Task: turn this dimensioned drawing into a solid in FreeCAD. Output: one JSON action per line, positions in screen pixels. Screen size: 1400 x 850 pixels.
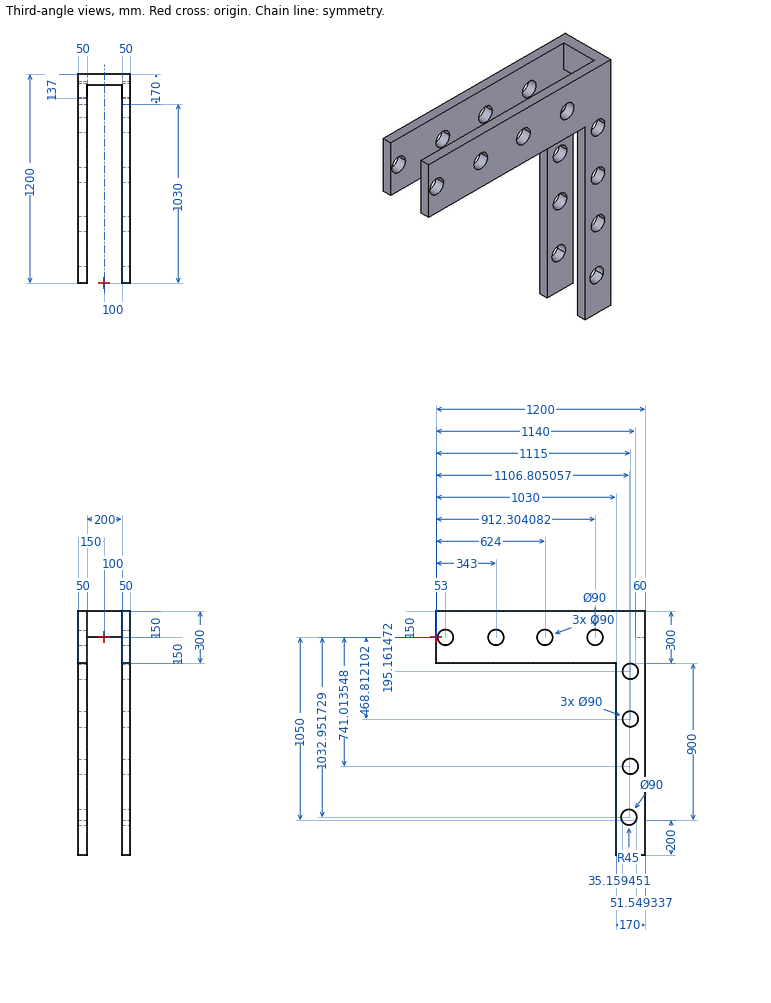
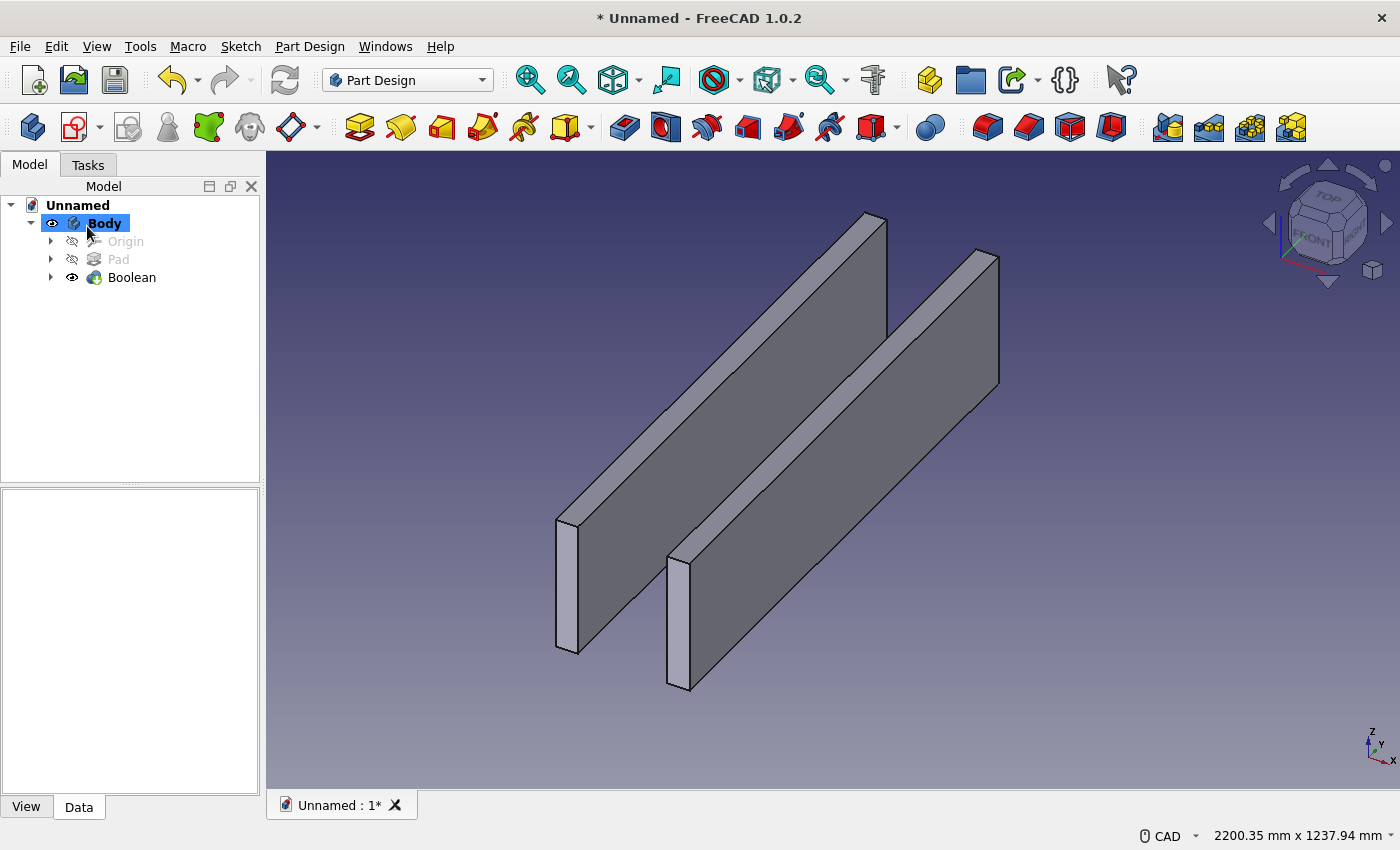
{"action": "left_click", "coordinate": [51, 241]}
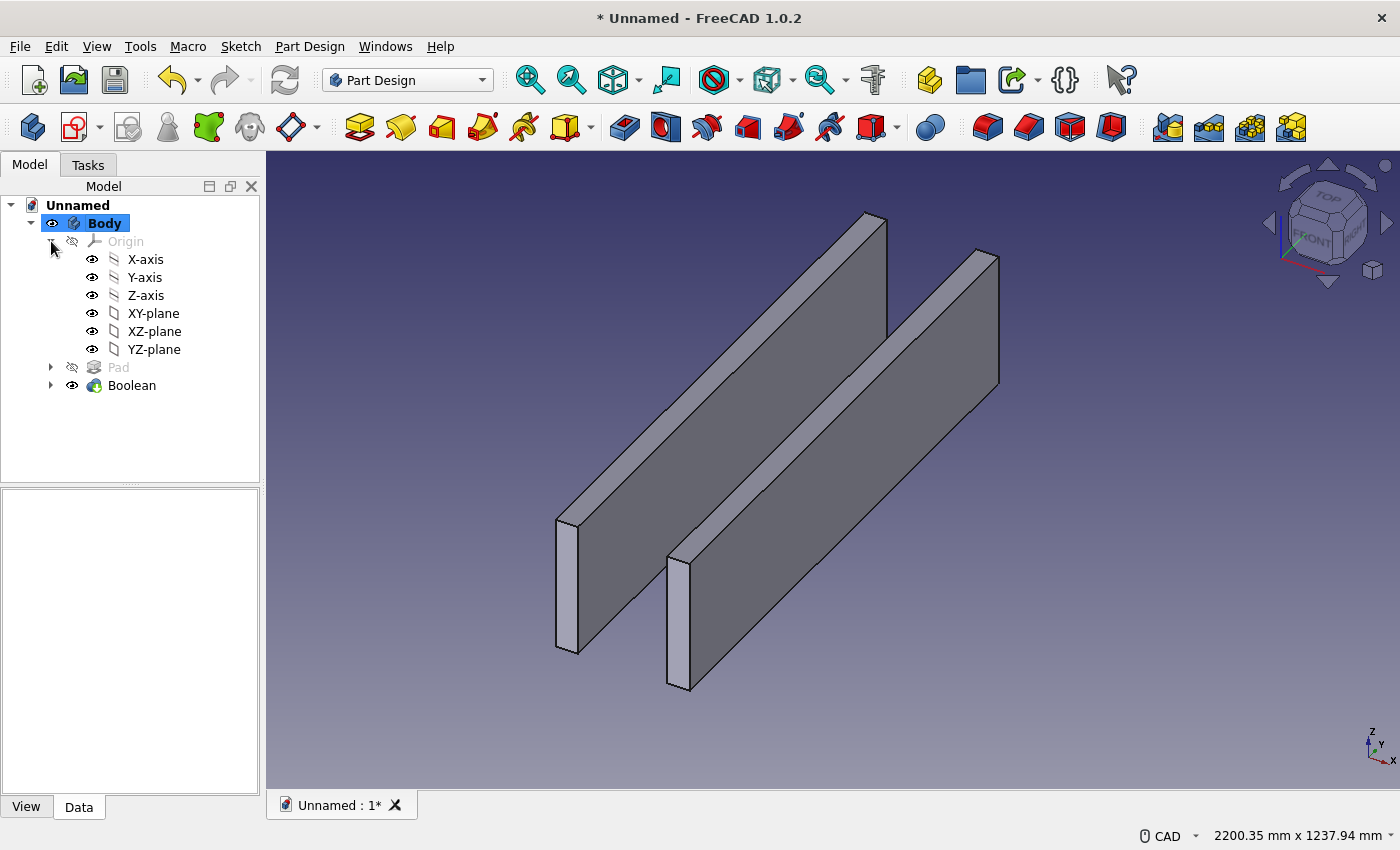
{"action": "left_click", "coordinate": [137, 349]}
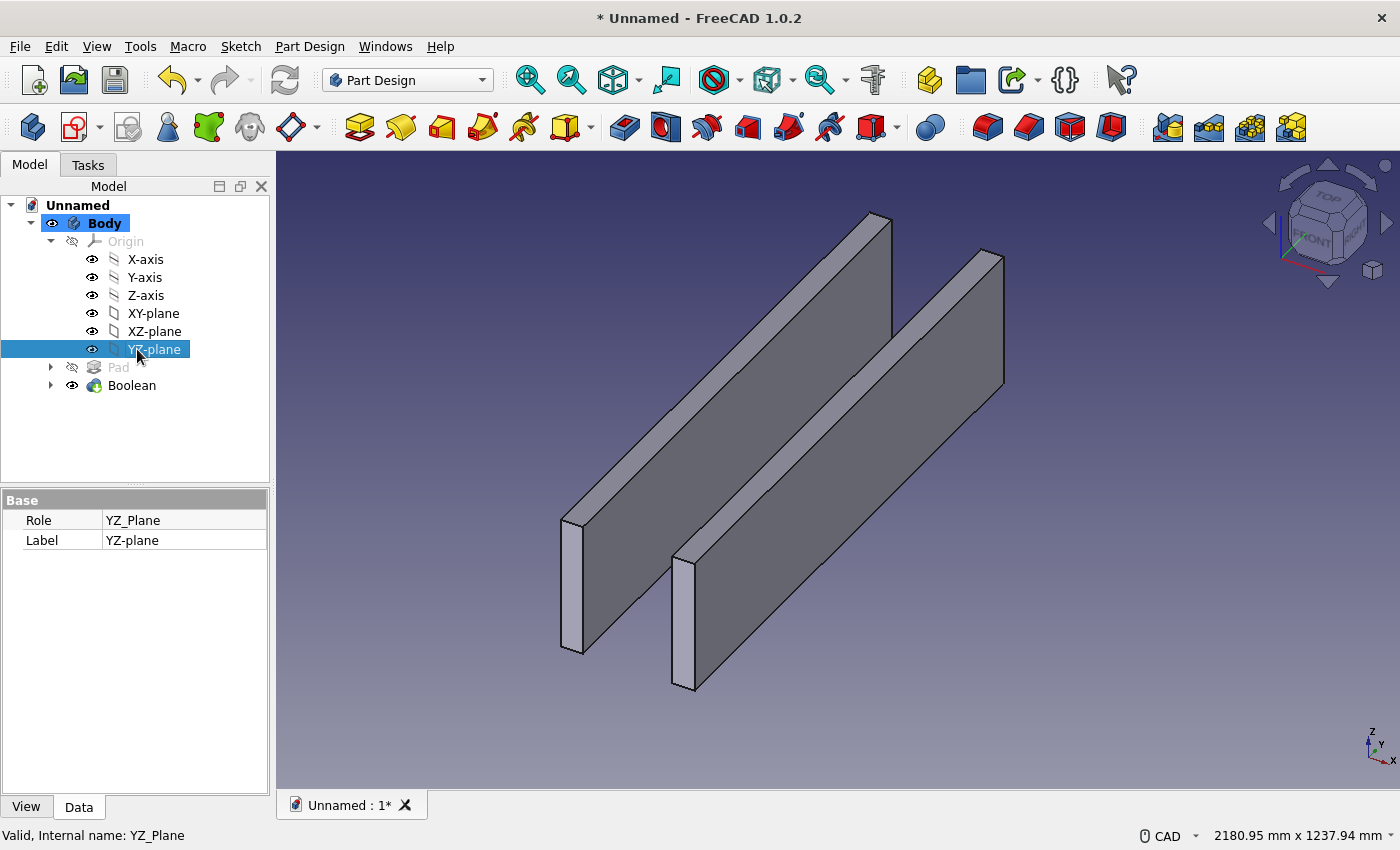
{"action": "left_click", "coordinate": [290, 128]}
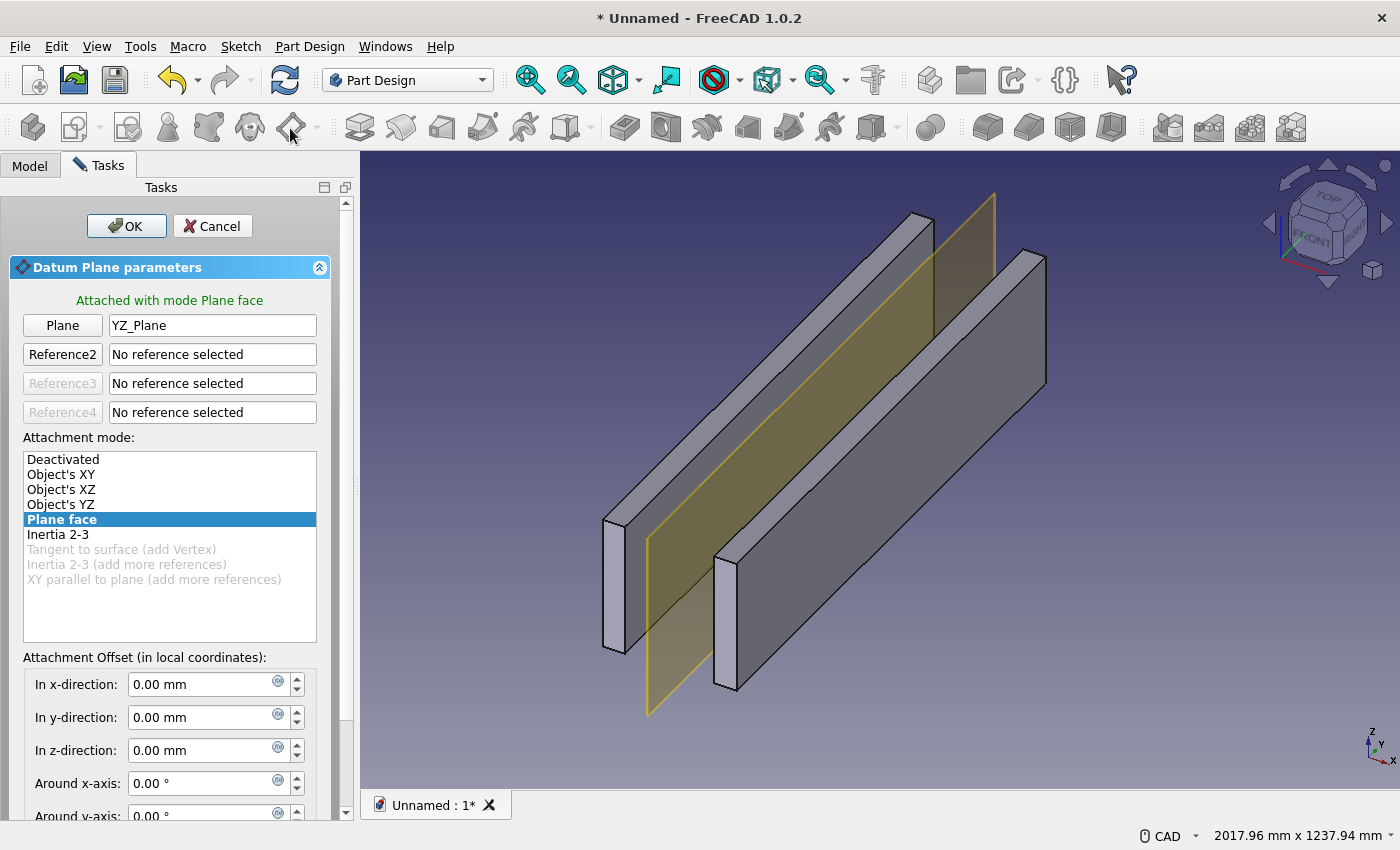
{"action": "triple_click", "coordinate": [210, 750]}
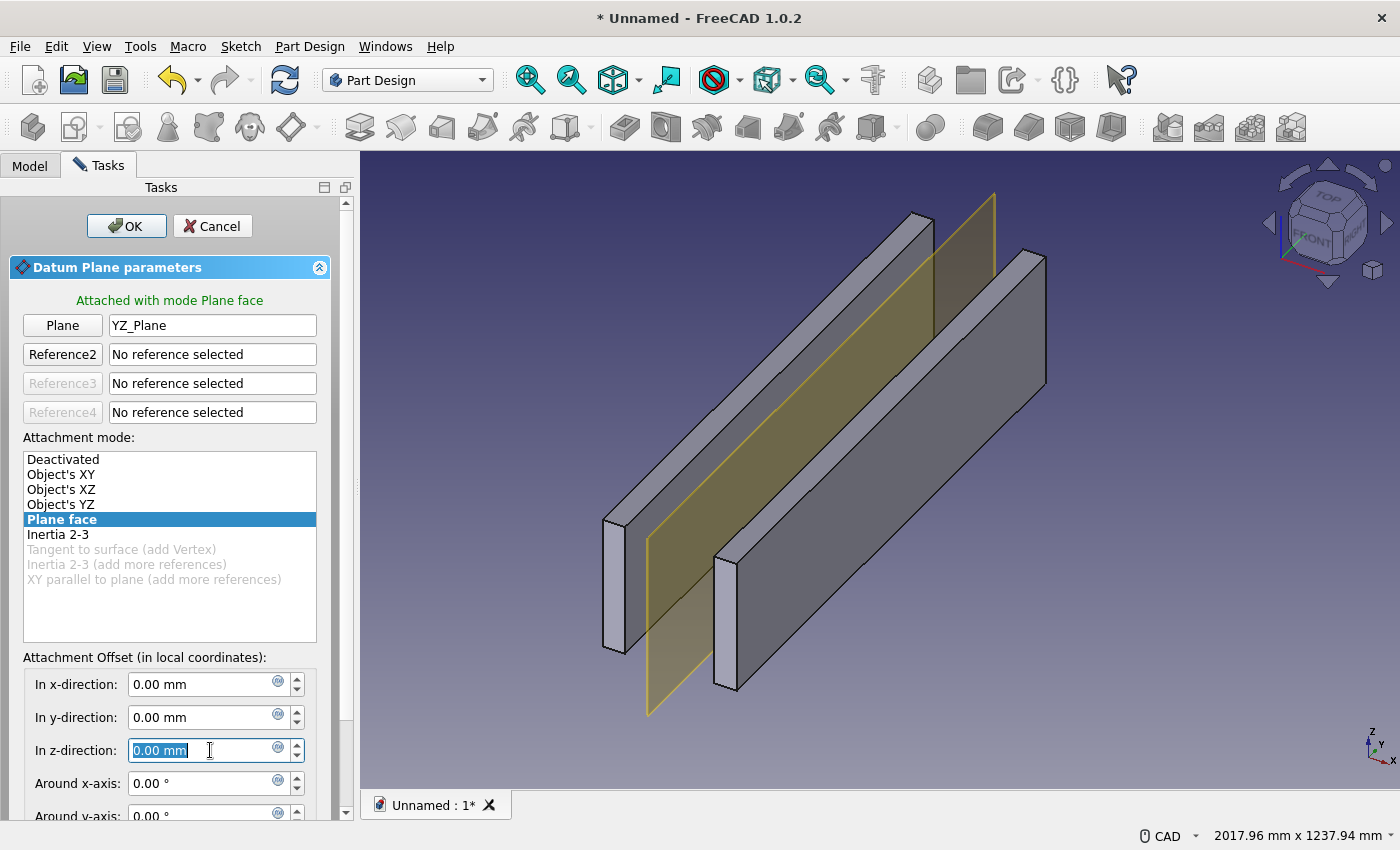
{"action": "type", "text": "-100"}
{"action": "key", "text": "Tab"}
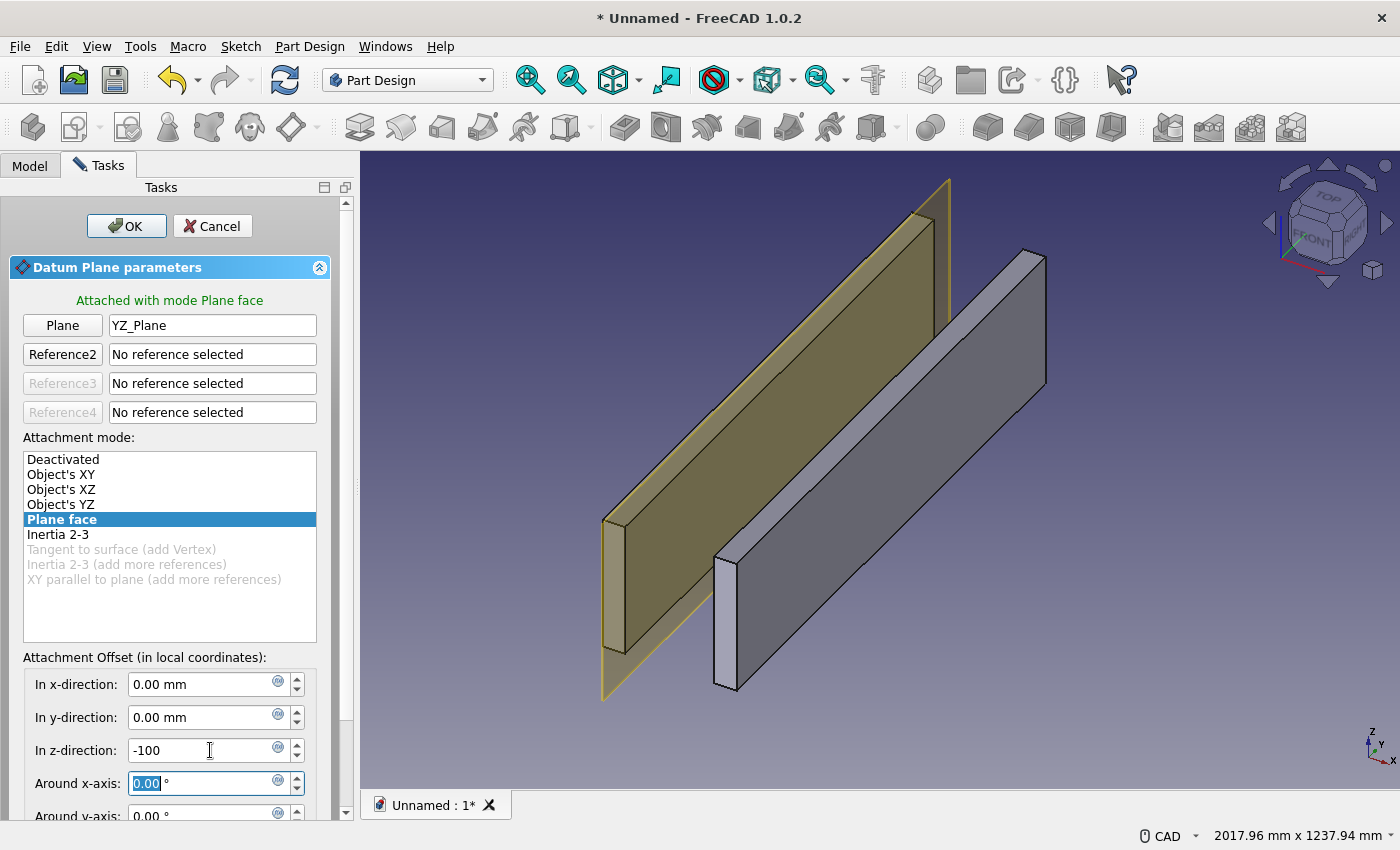
{"action": "left_click", "coordinate": [127, 226]}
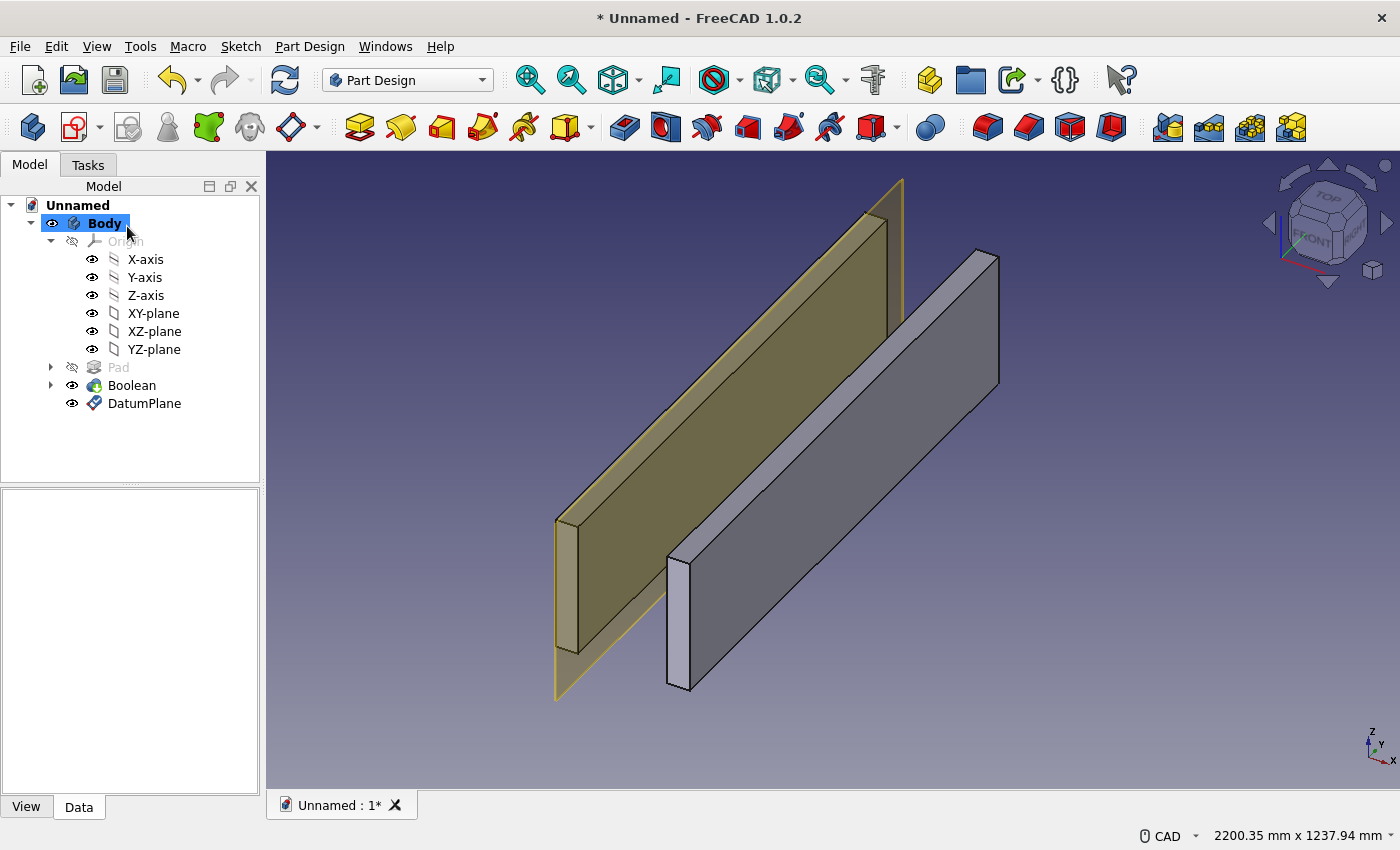
{"action": "left_click", "coordinate": [117, 403]}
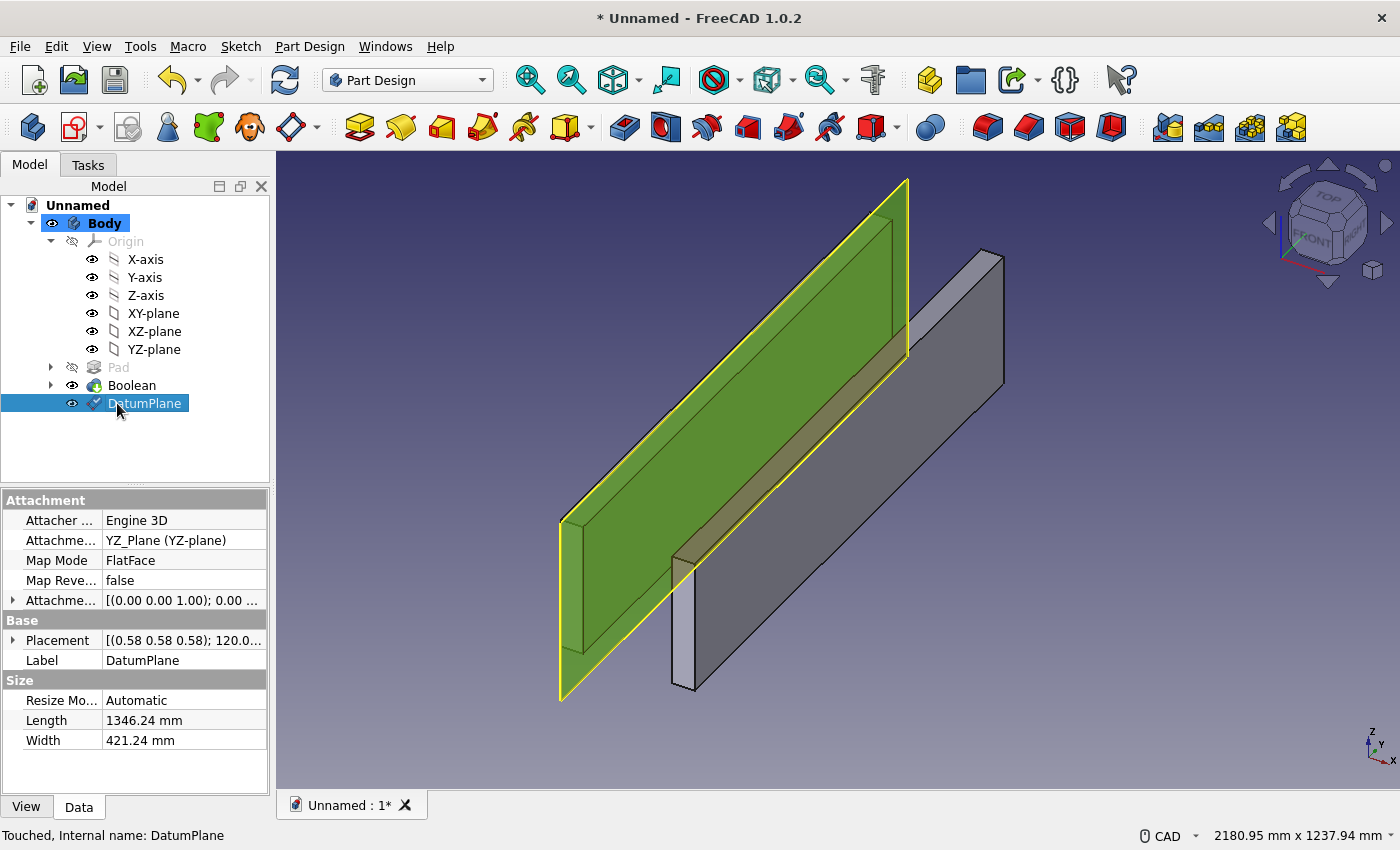
{"action": "left_click", "coordinate": [74, 128]}